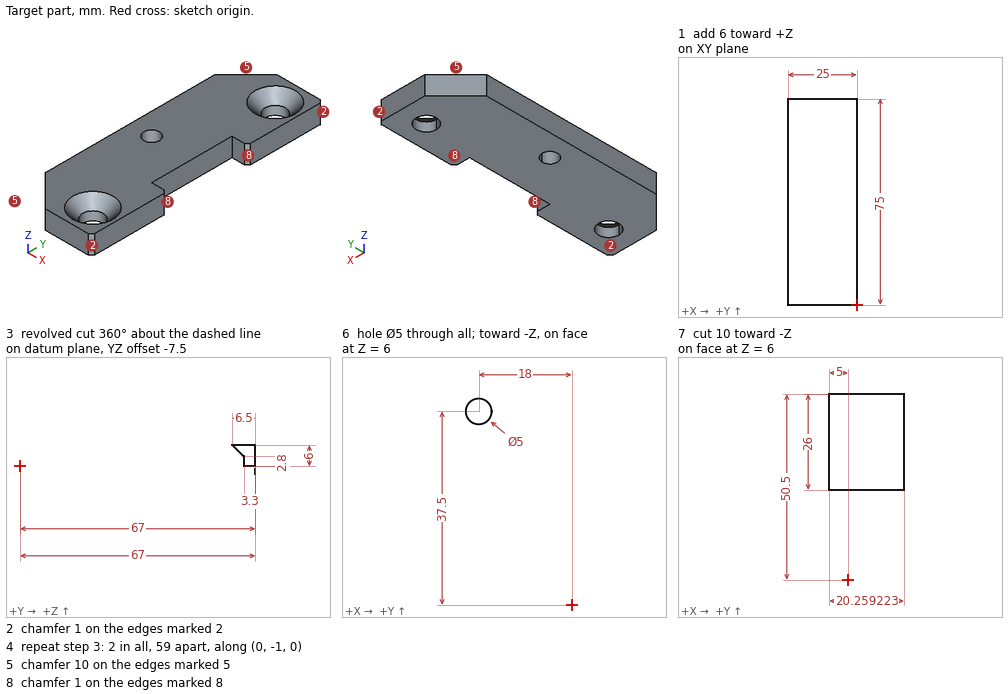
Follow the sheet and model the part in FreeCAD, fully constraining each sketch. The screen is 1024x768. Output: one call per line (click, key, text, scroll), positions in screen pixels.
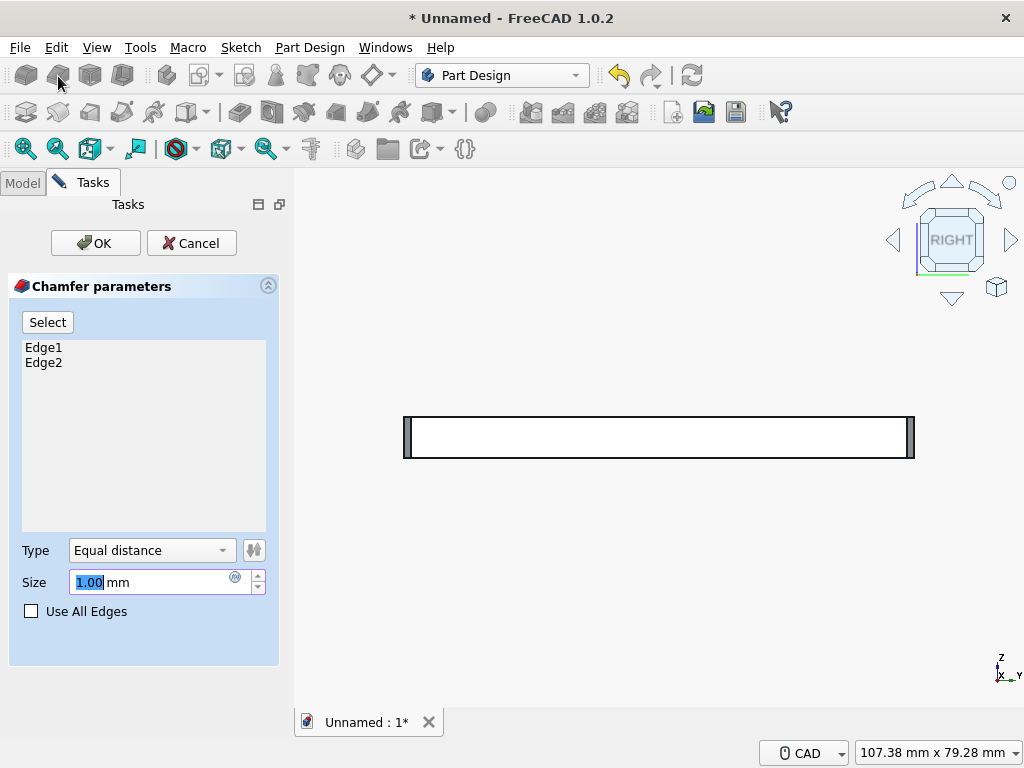
text(1)
key(Tab)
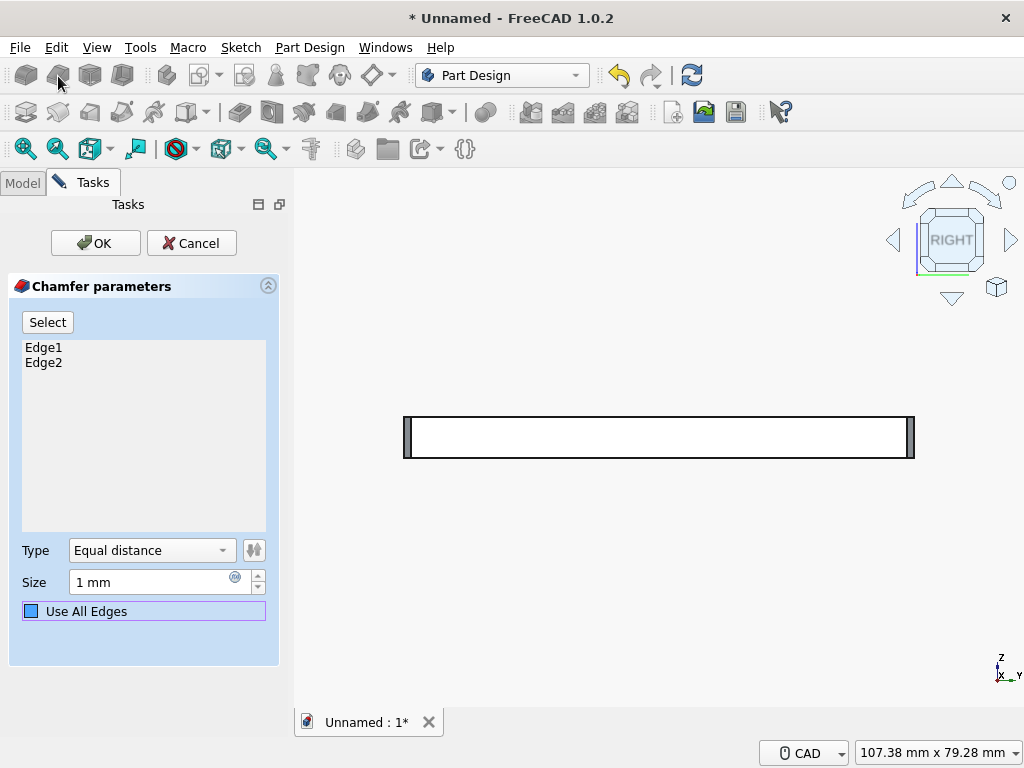
click(96, 243)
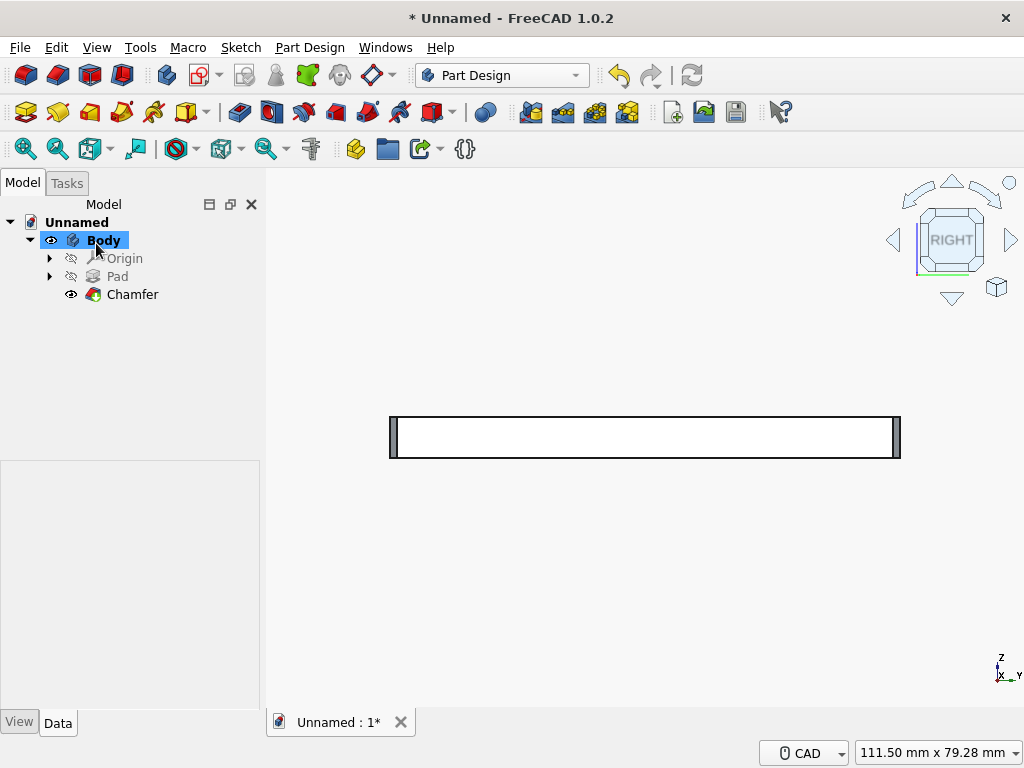
click(50, 258)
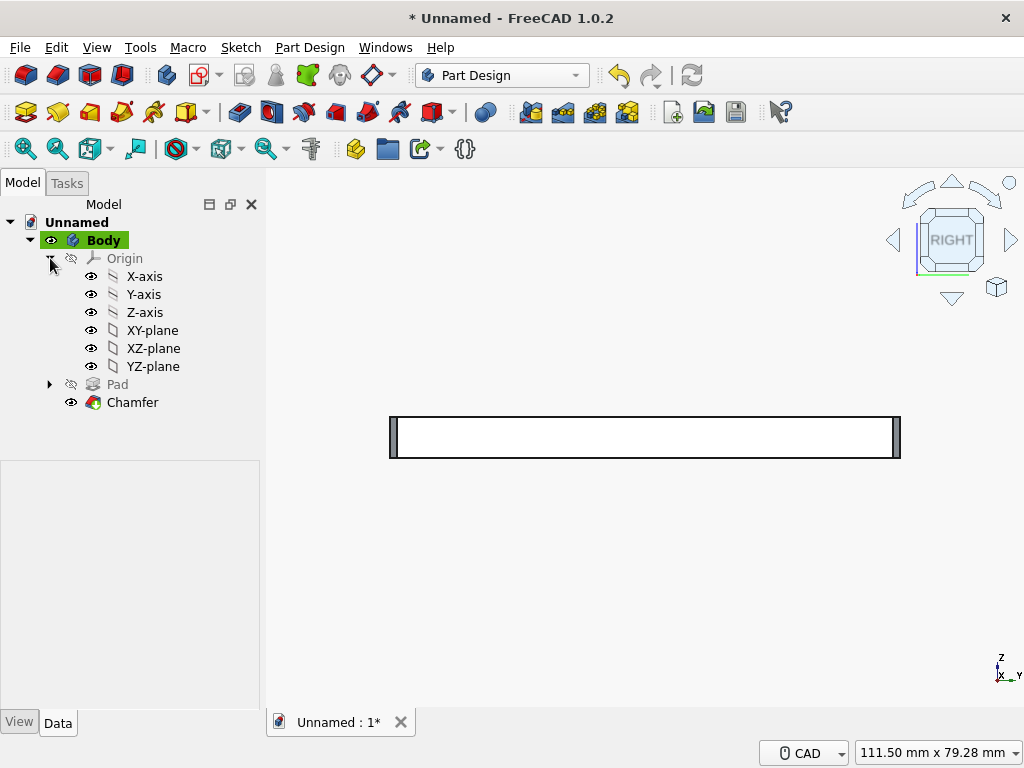
click(136, 366)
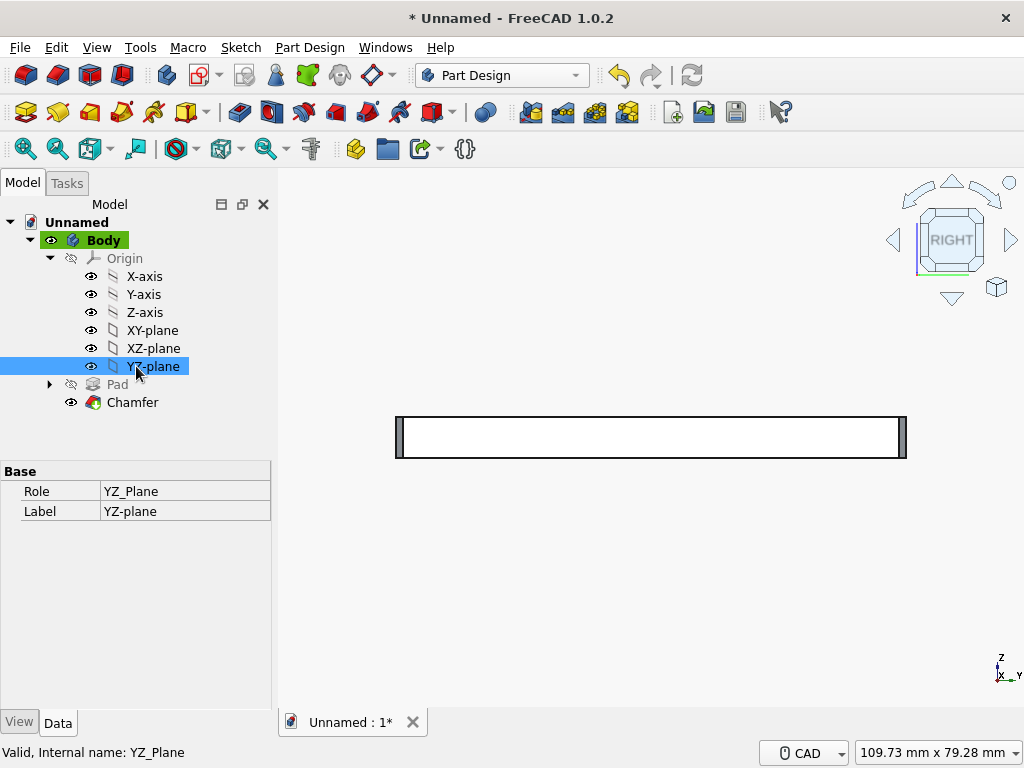
click(372, 76)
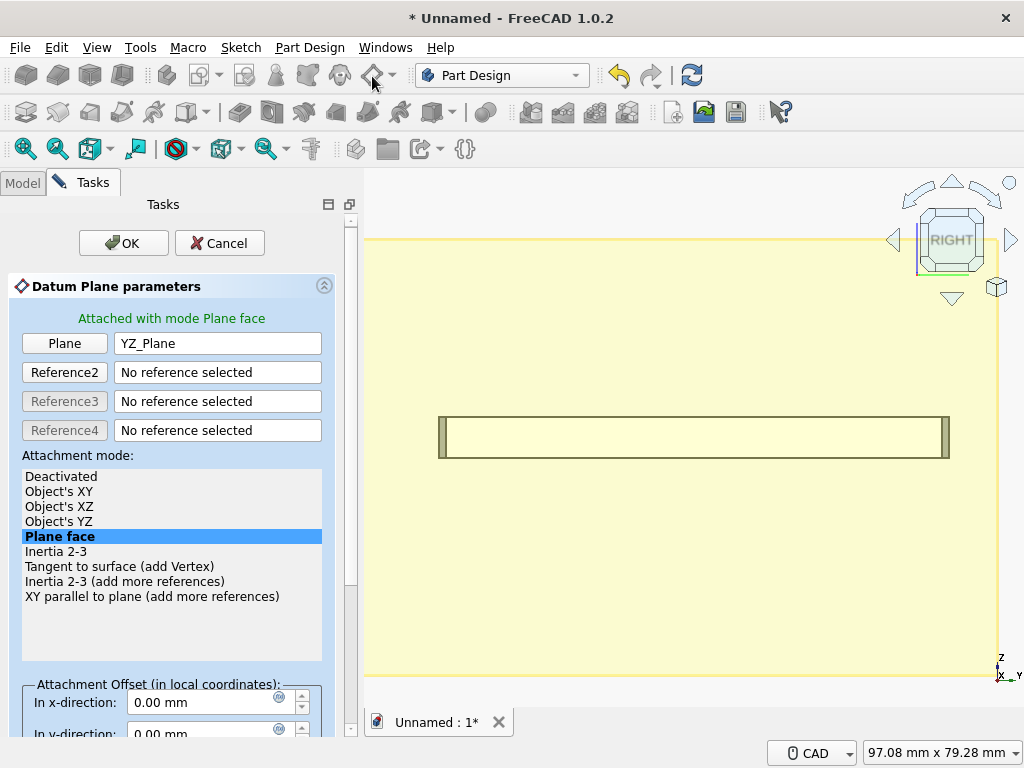
scroll(351, 475, down, 2)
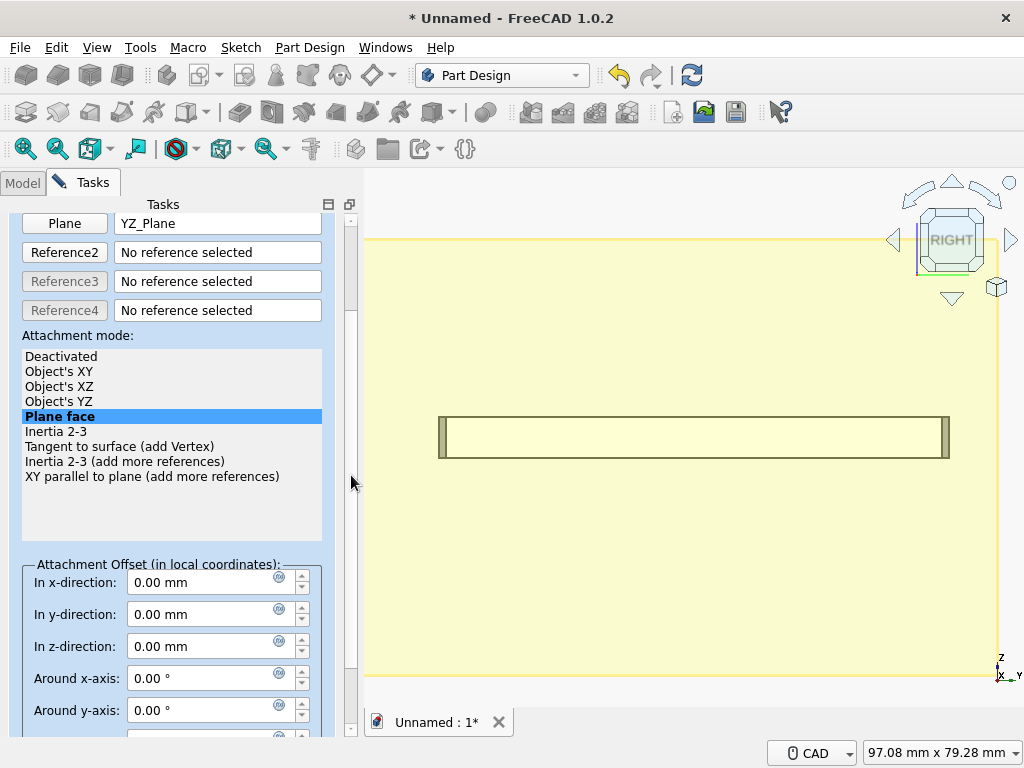
triple_click(210, 646)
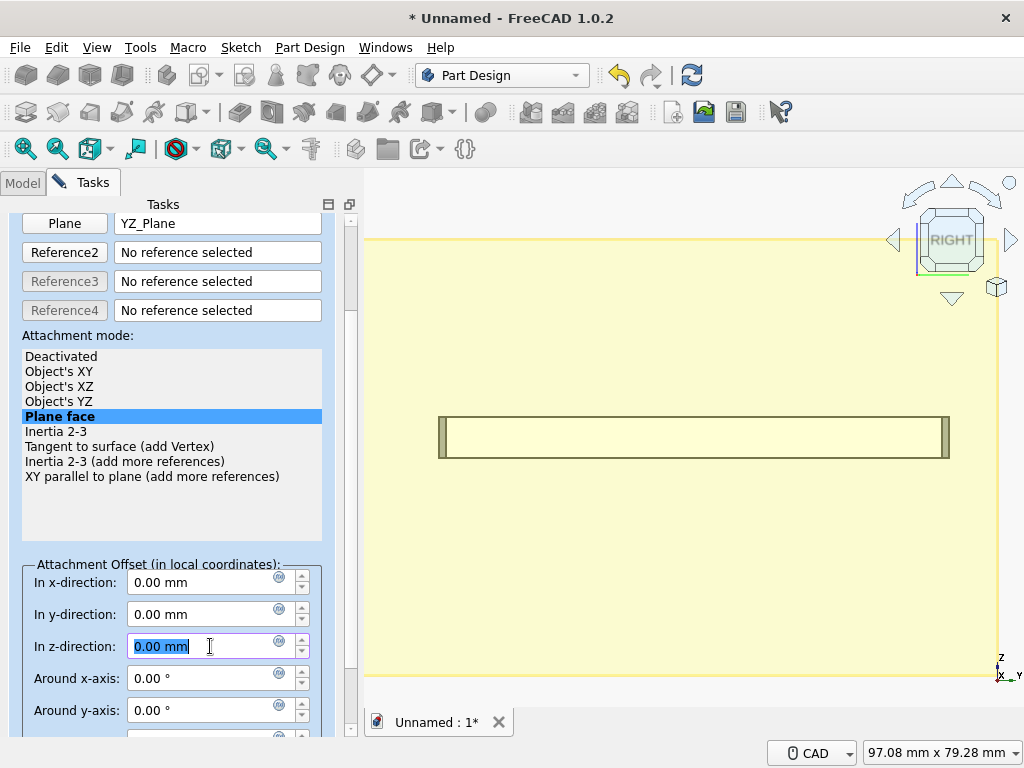
text(-7.5)
key(Tab)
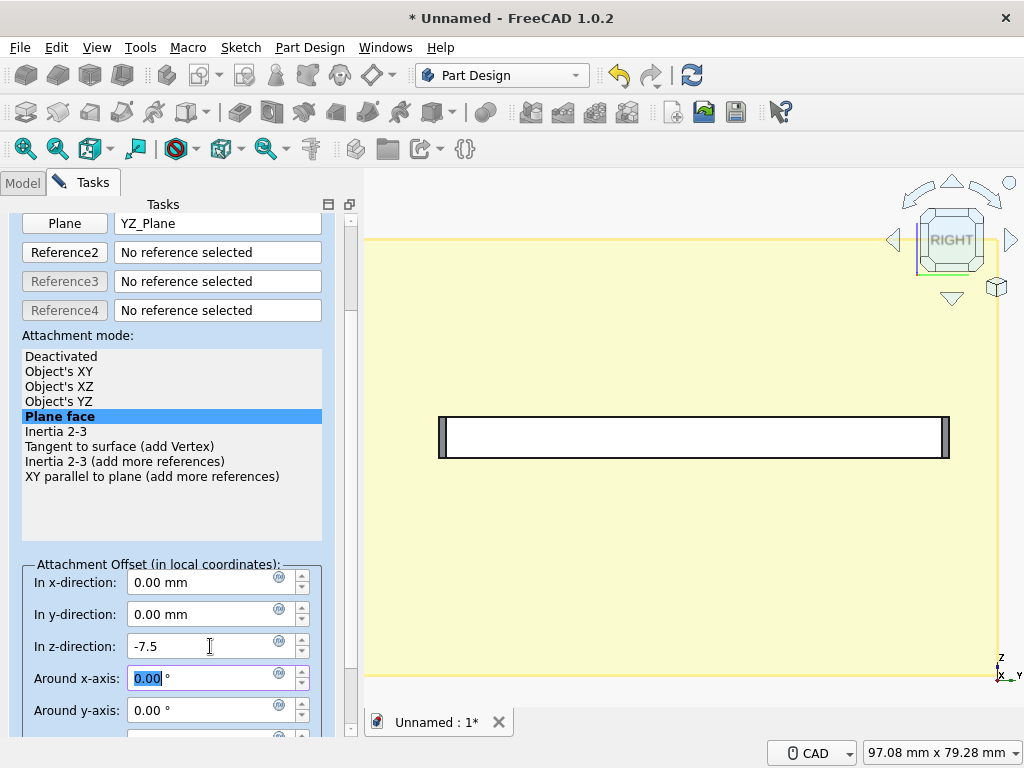
scroll(351, 475, up, 3)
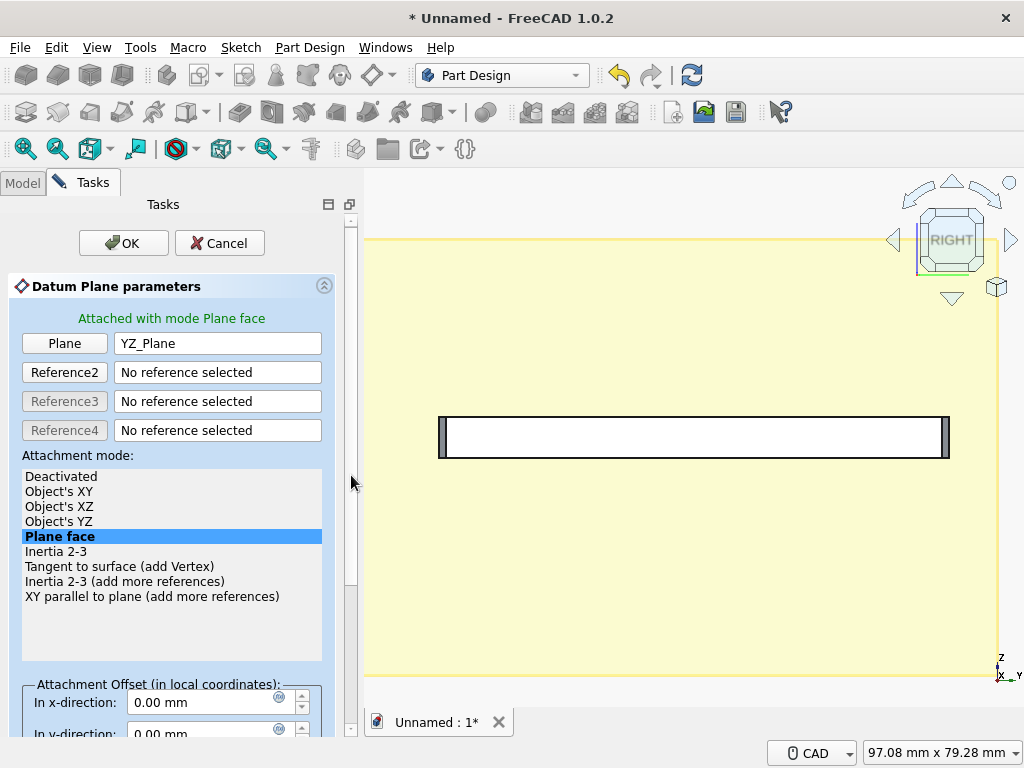
click(124, 243)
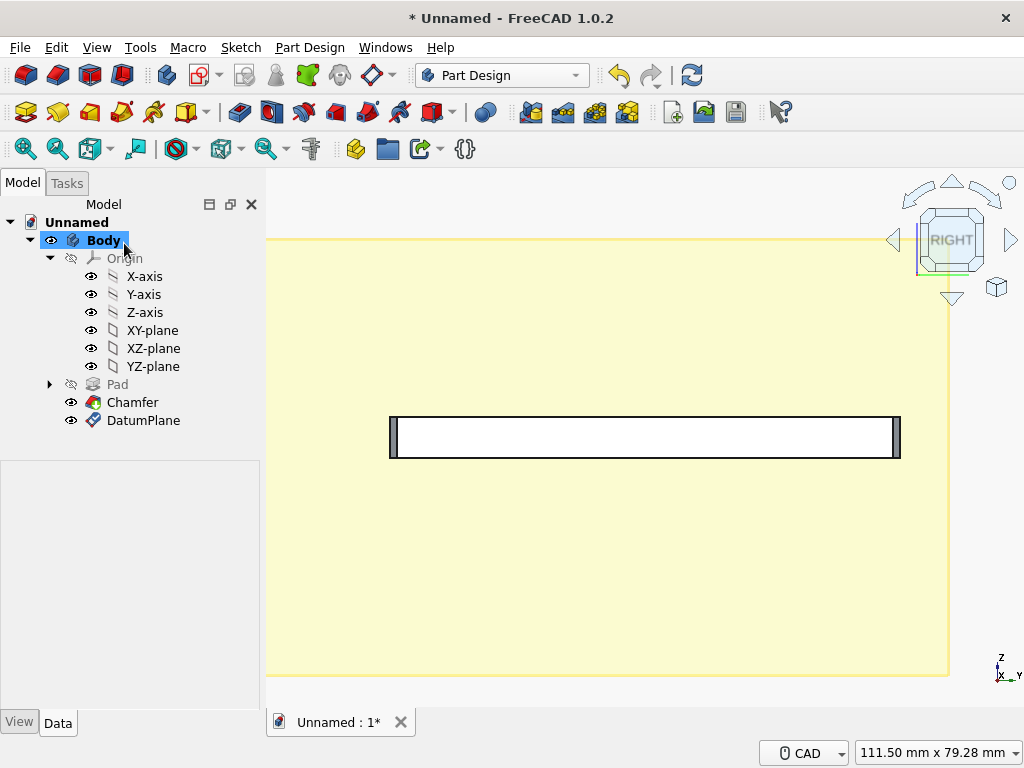
click(116, 420)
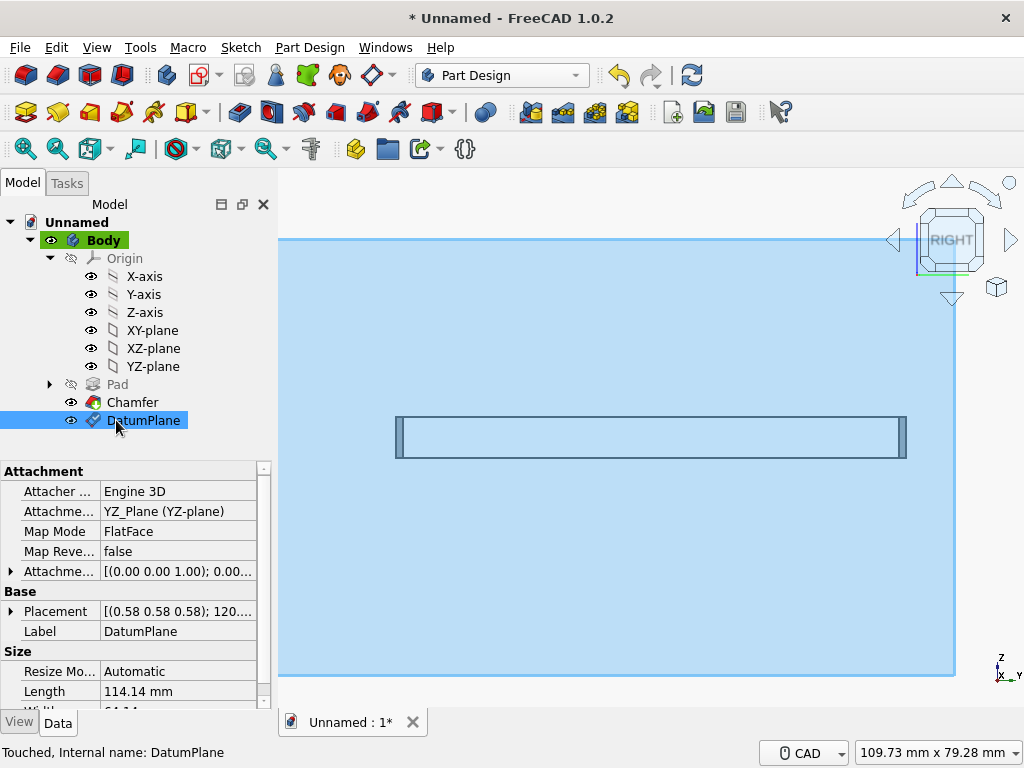
click(200, 76)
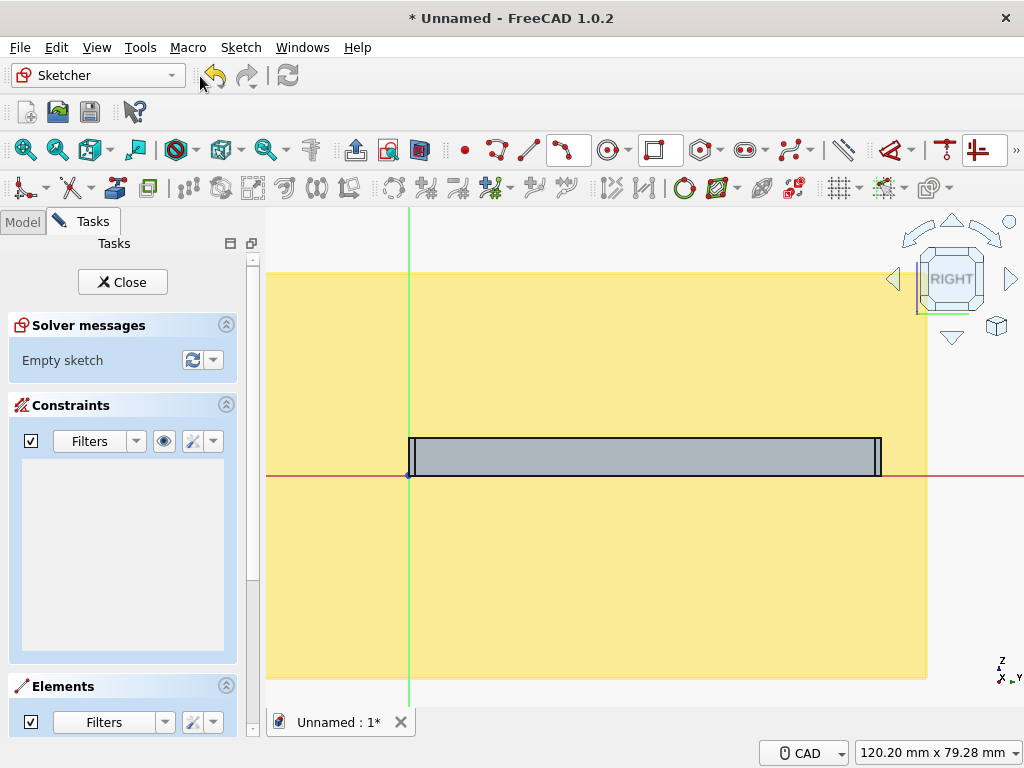
click(420, 150)